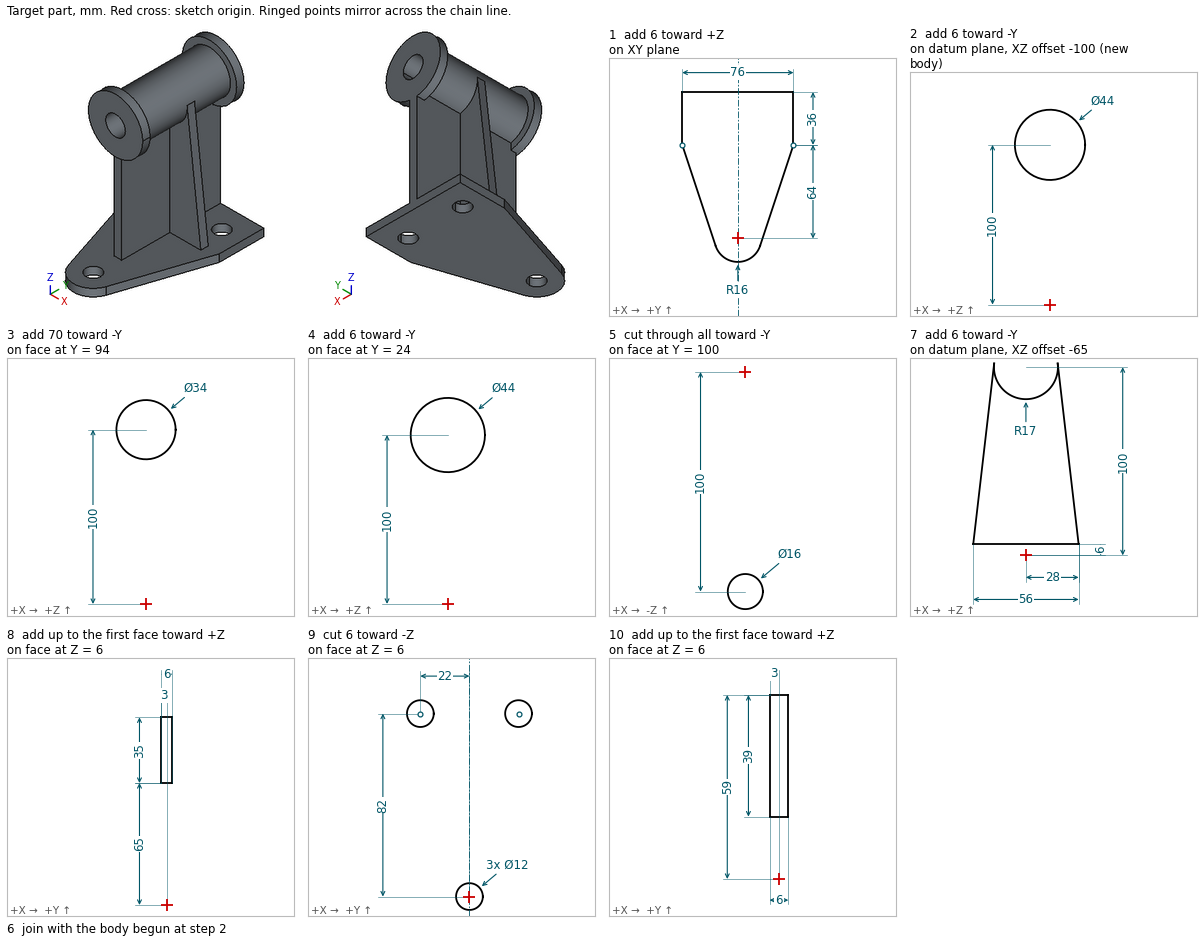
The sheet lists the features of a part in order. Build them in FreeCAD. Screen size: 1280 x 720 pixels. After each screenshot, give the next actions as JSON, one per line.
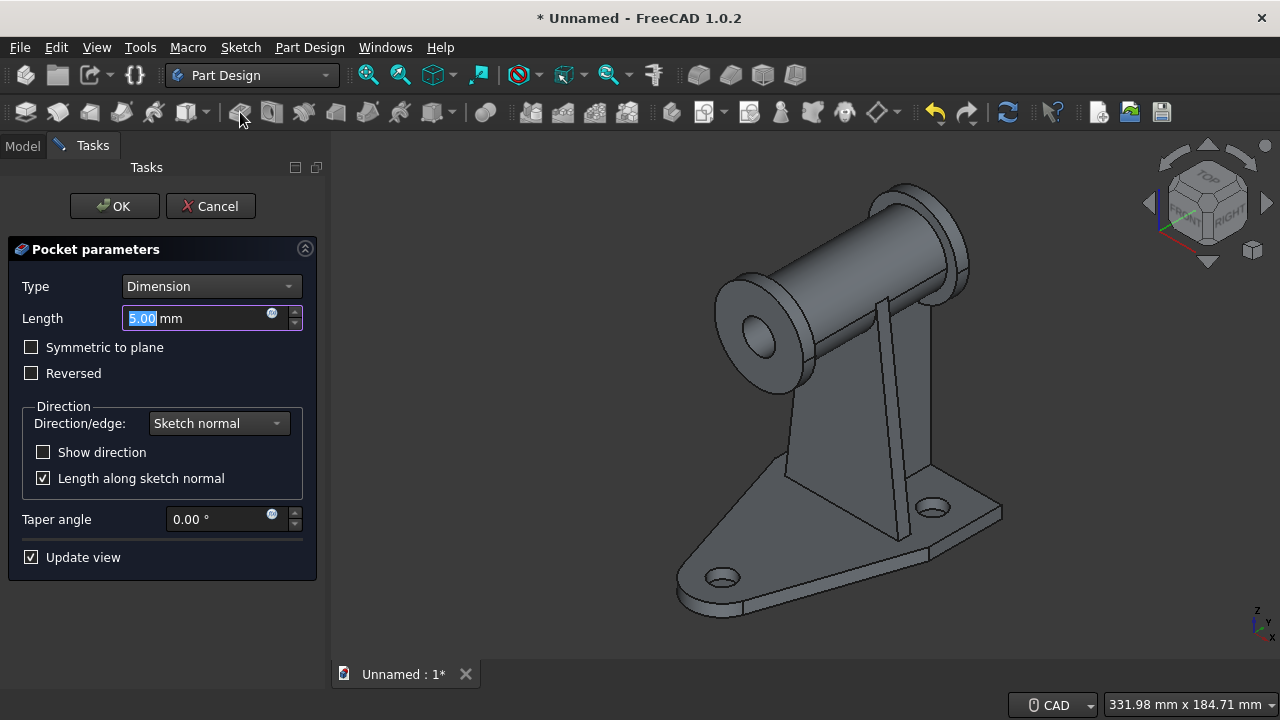
{"action": "type", "text": "6"}
{"action": "key", "text": "Tab"}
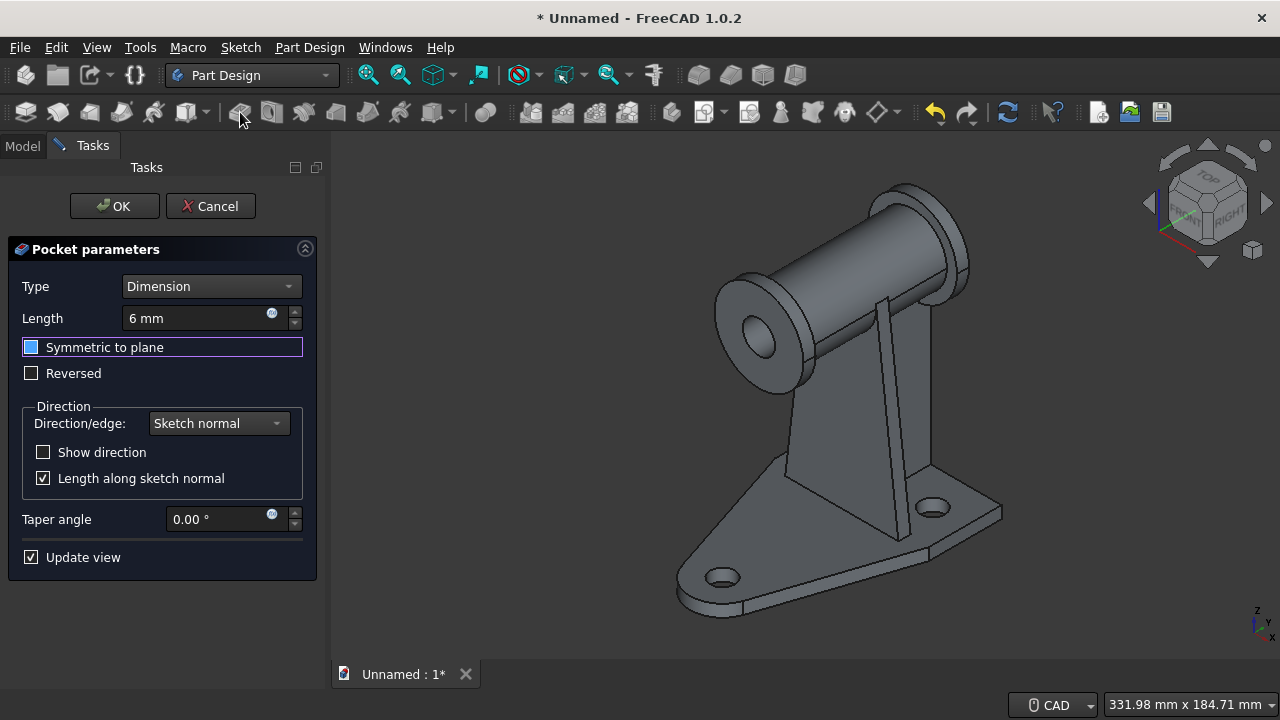
{"action": "left_click", "coordinate": [115, 206]}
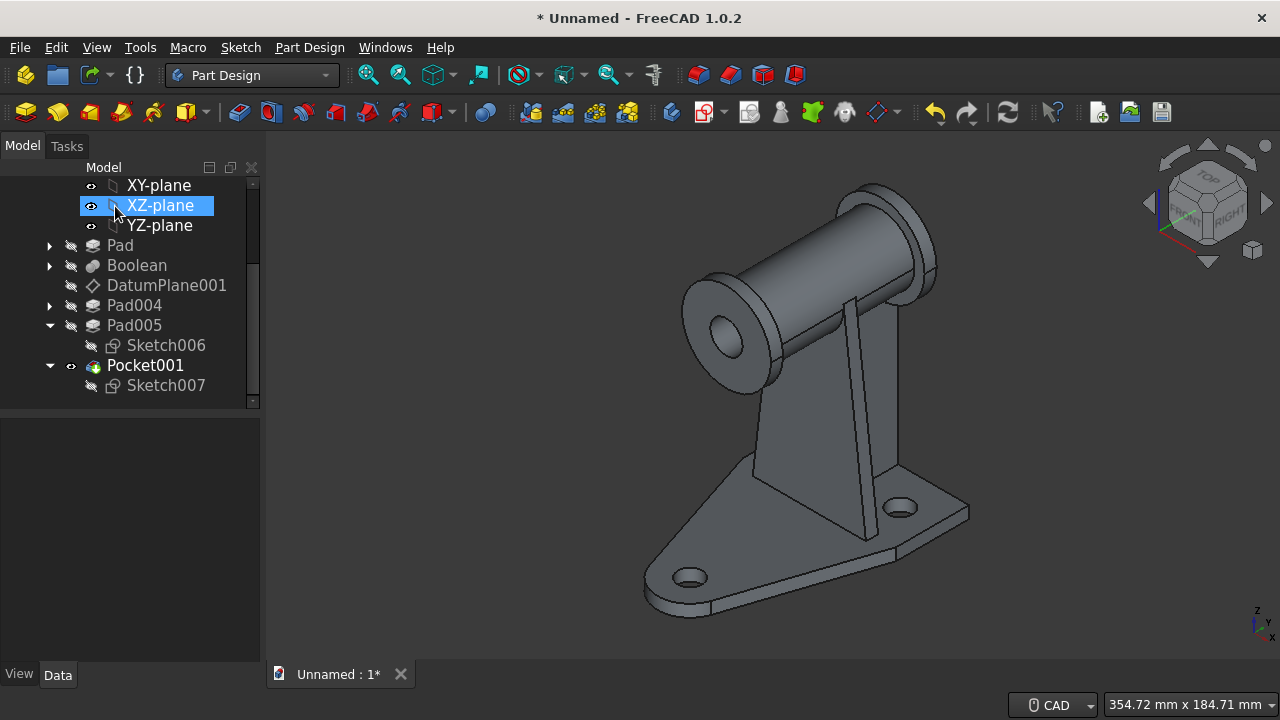
{"action": "left_click", "coordinate": [819, 553]}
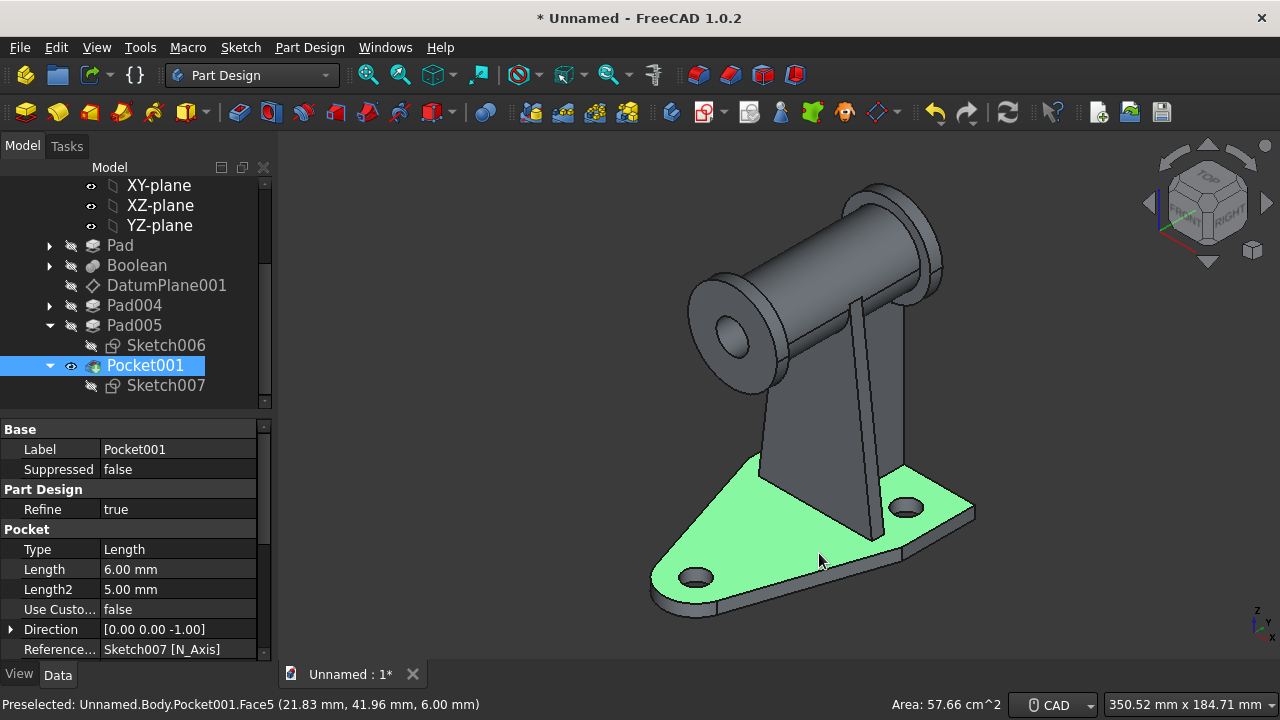
{"action": "left_click", "coordinate": [704, 112]}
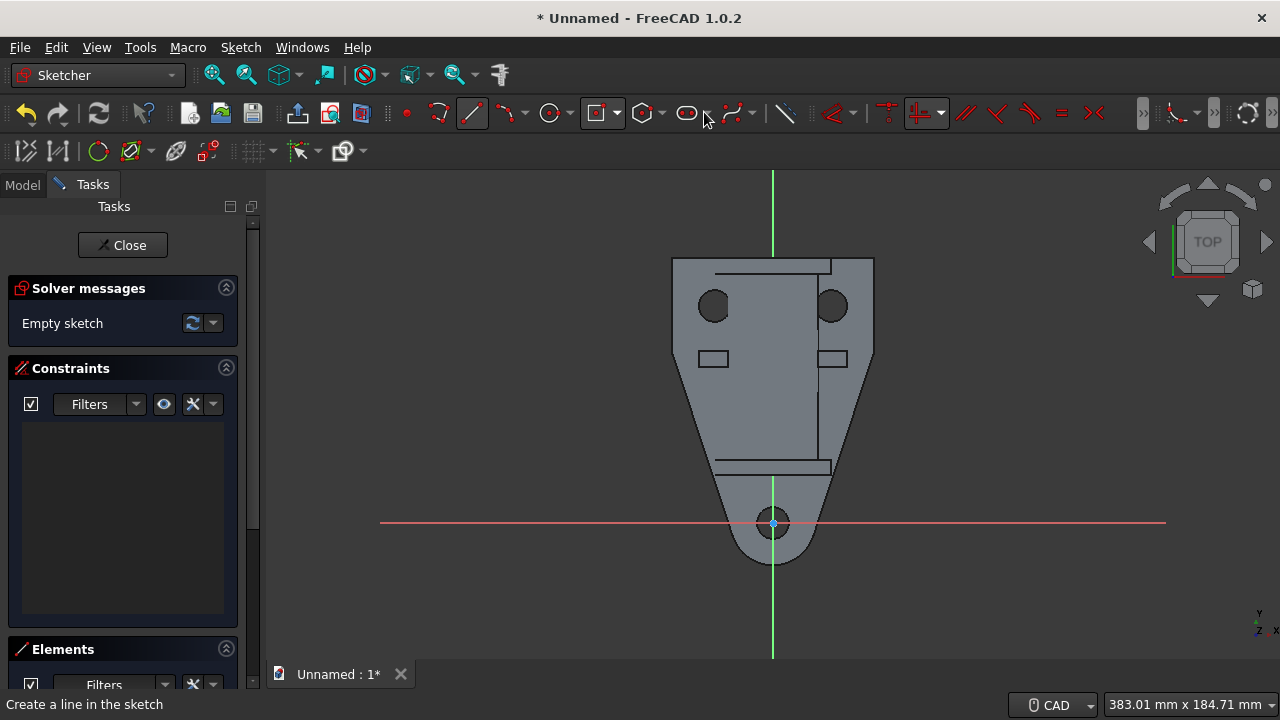
{"action": "scroll", "coordinate": [856, 482], "scroll_direction": "up", "scroll_amount": 3}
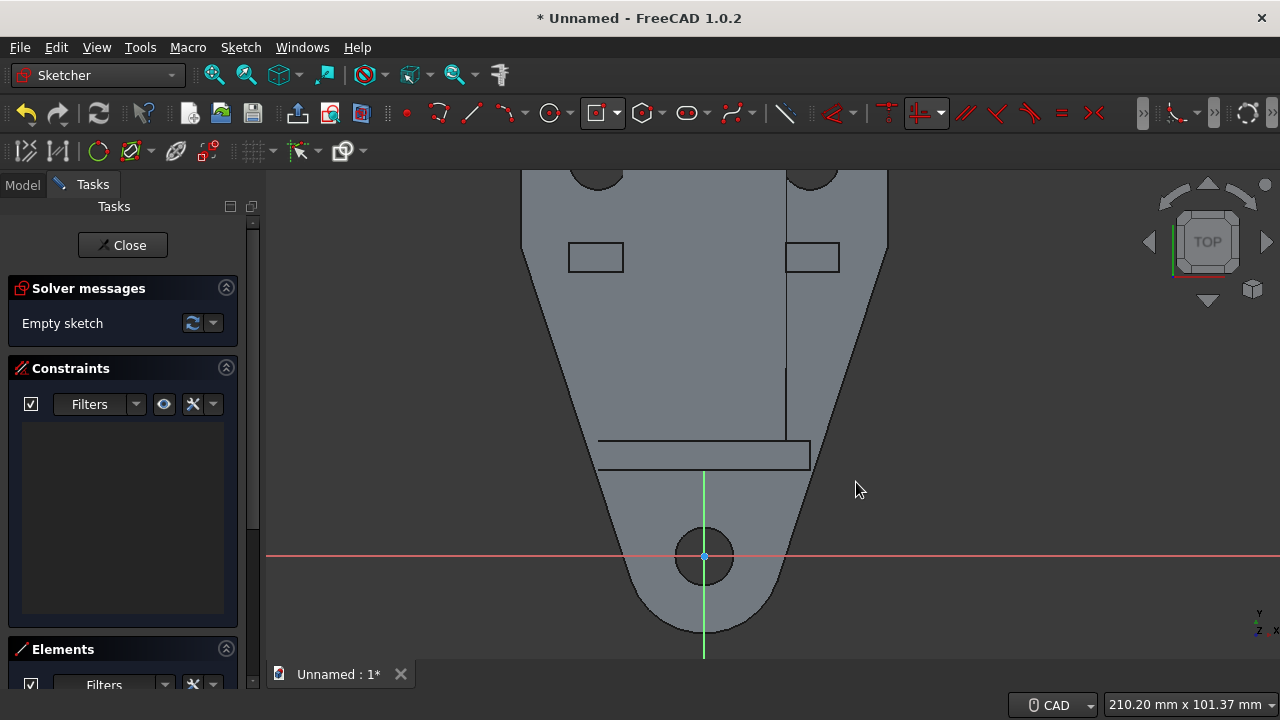
{"action": "key", "text": "g r"}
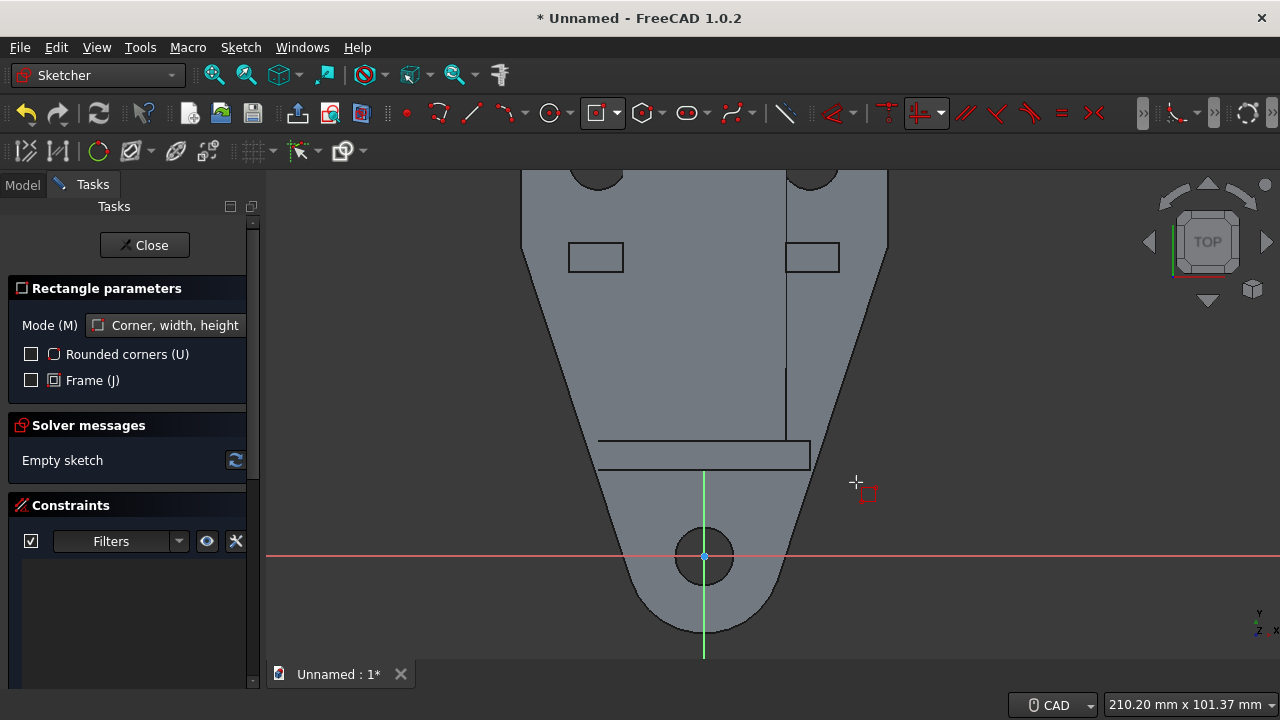
{"action": "left_click", "coordinate": [690, 272]}
{"action": "left_click", "coordinate": [719, 460]}
{"action": "key", "text": "Escape"}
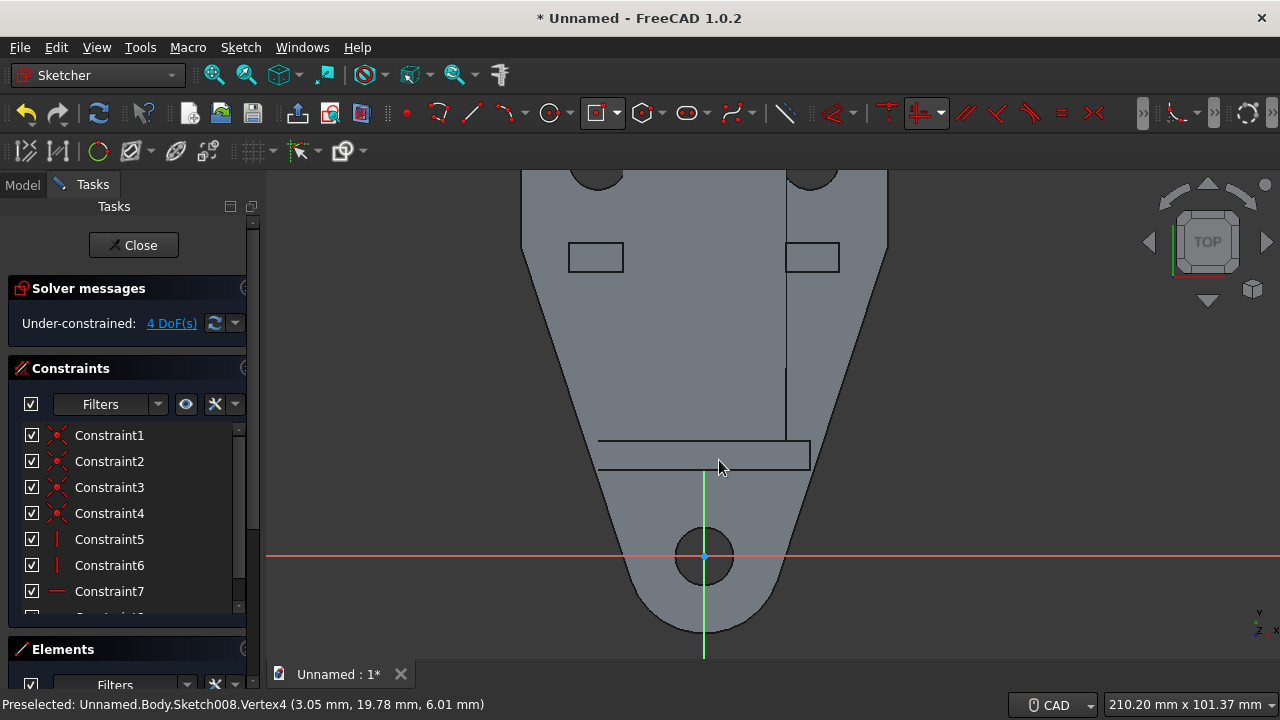
{"action": "key", "text": "d"}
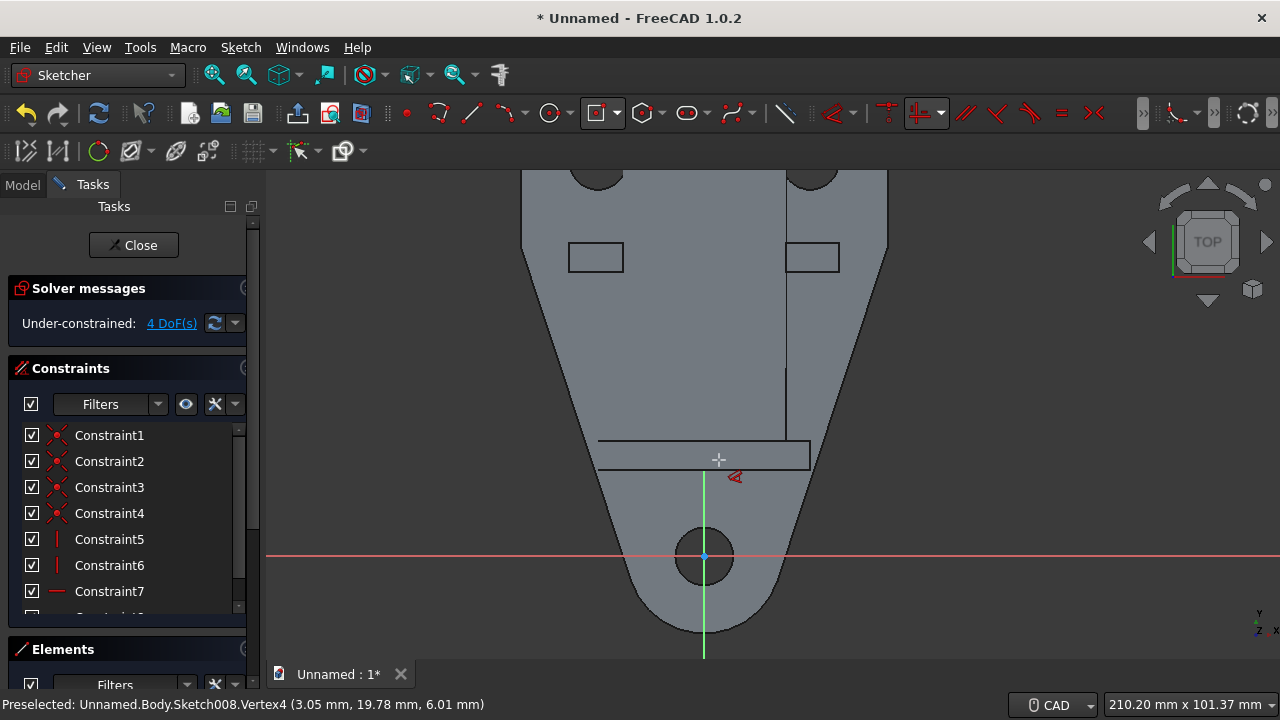
{"action": "scroll", "coordinate": [702, 461], "scroll_direction": "up", "scroll_amount": 2}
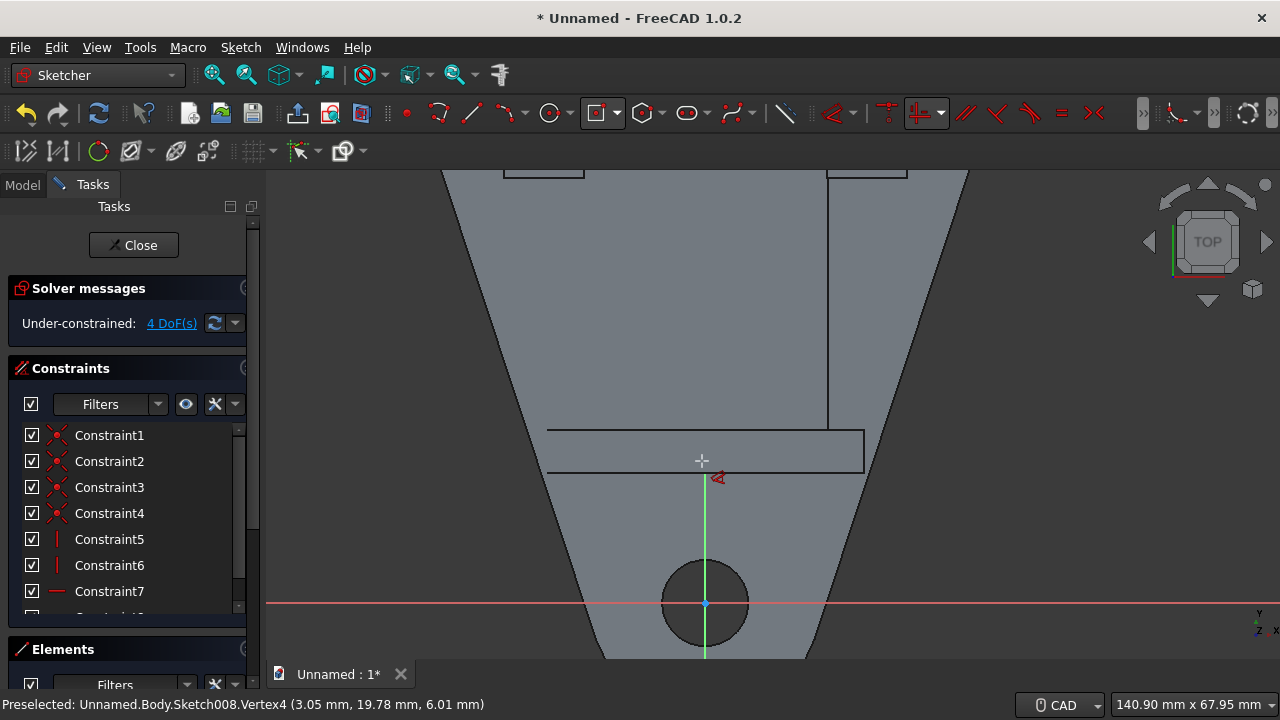
{"action": "left_click", "coordinate": [701, 461]}
{"action": "left_click", "coordinate": [690, 495]}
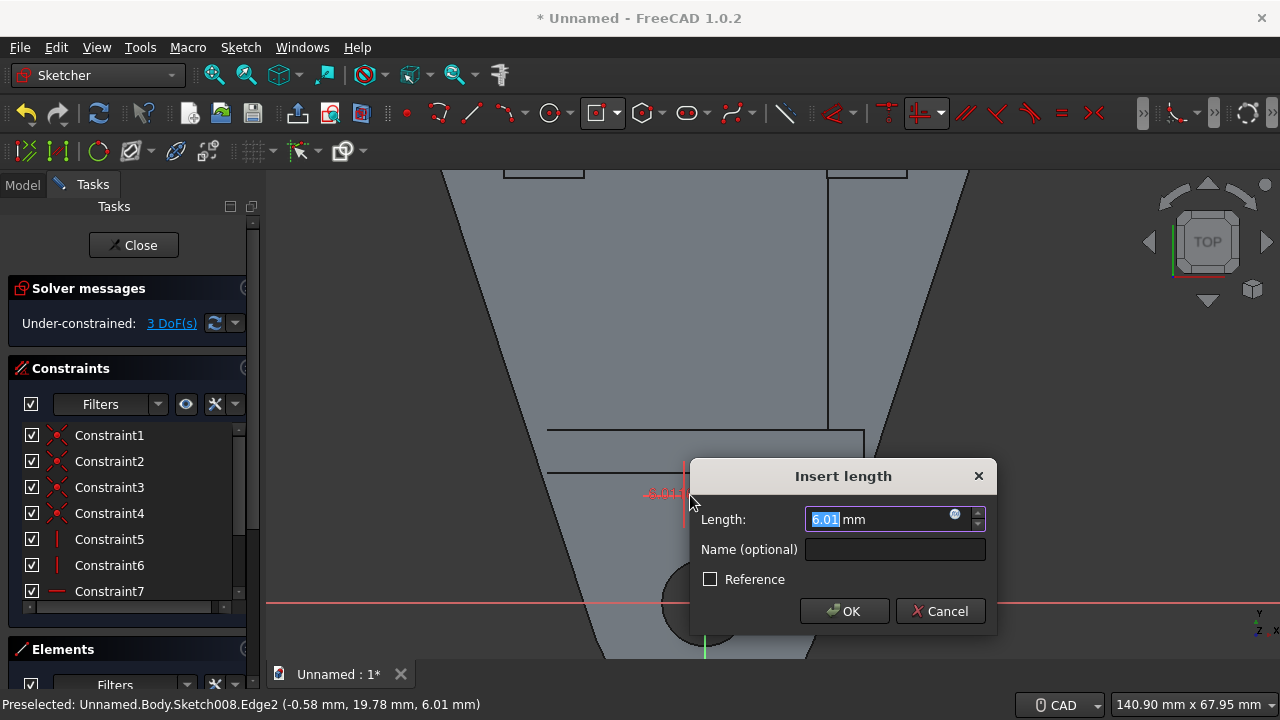
{"action": "type", "text": "6"}
{"action": "key", "text": "Return"}